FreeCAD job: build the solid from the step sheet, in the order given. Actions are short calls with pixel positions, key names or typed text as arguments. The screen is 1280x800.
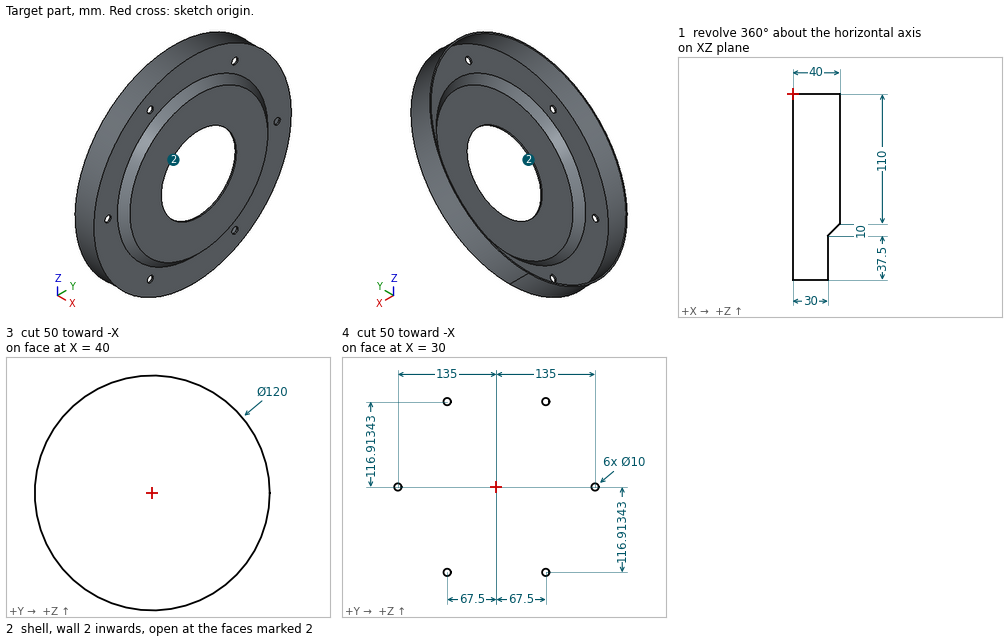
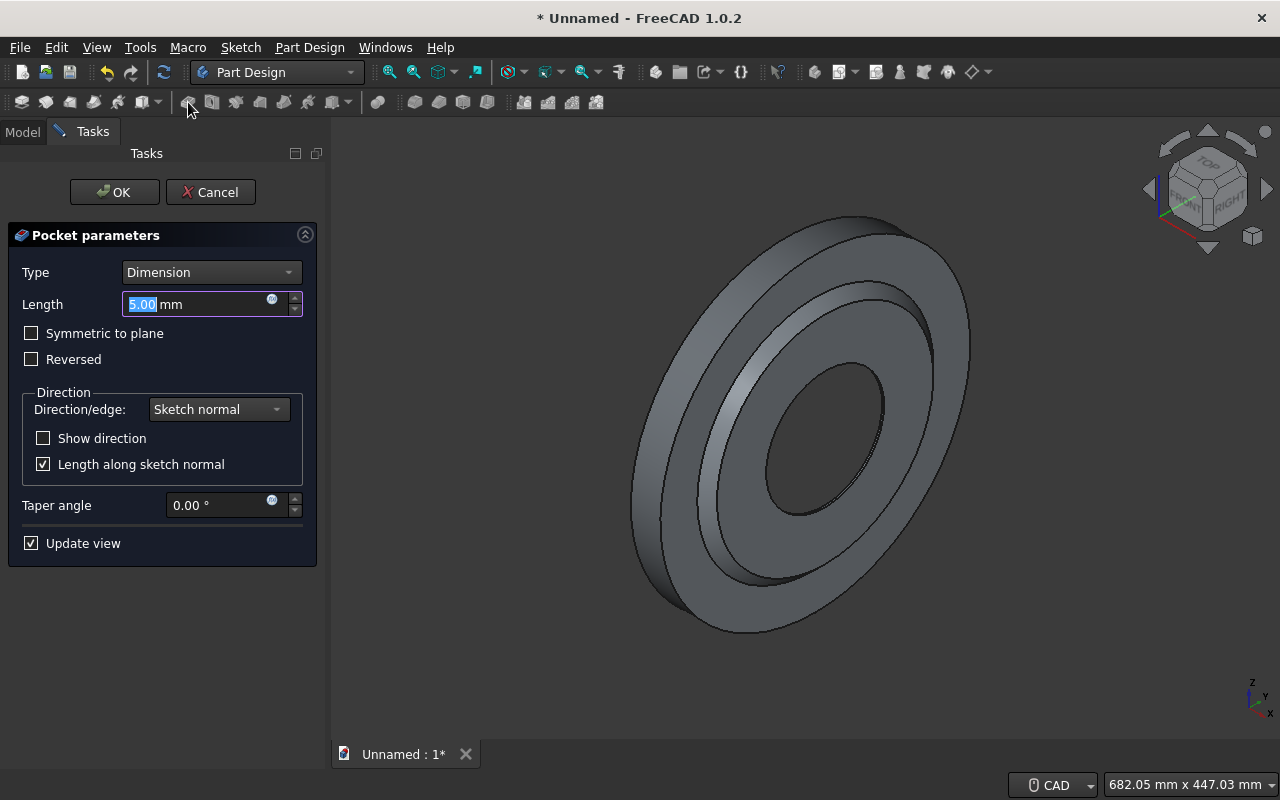
text(50)
key(Tab)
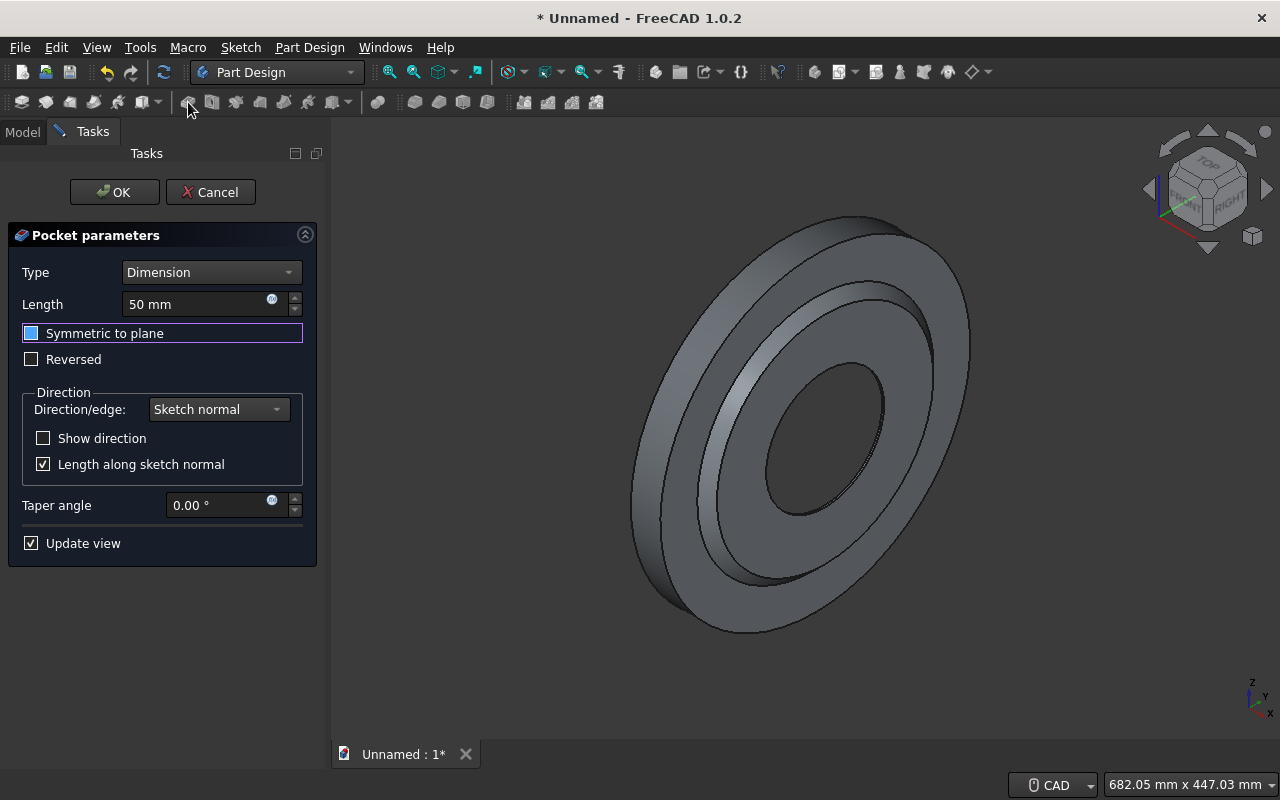
click(115, 192)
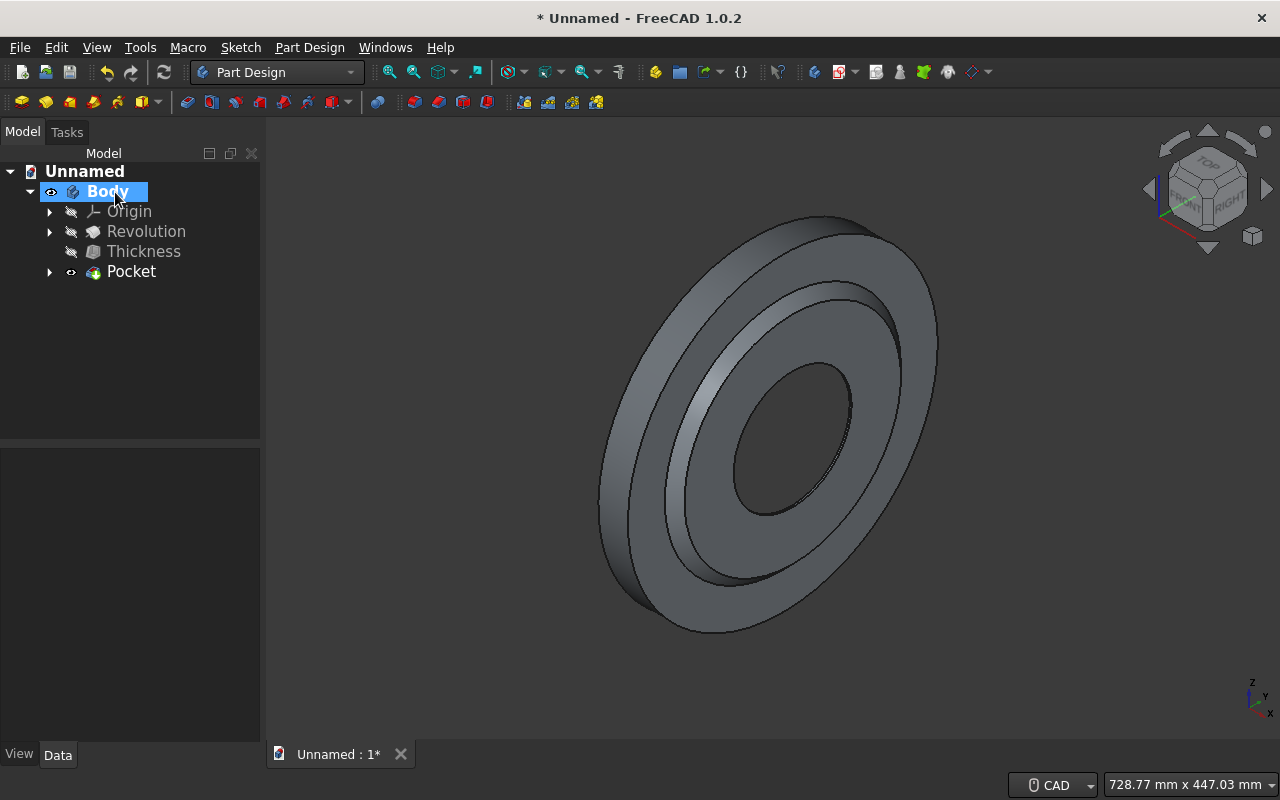
click(739, 611)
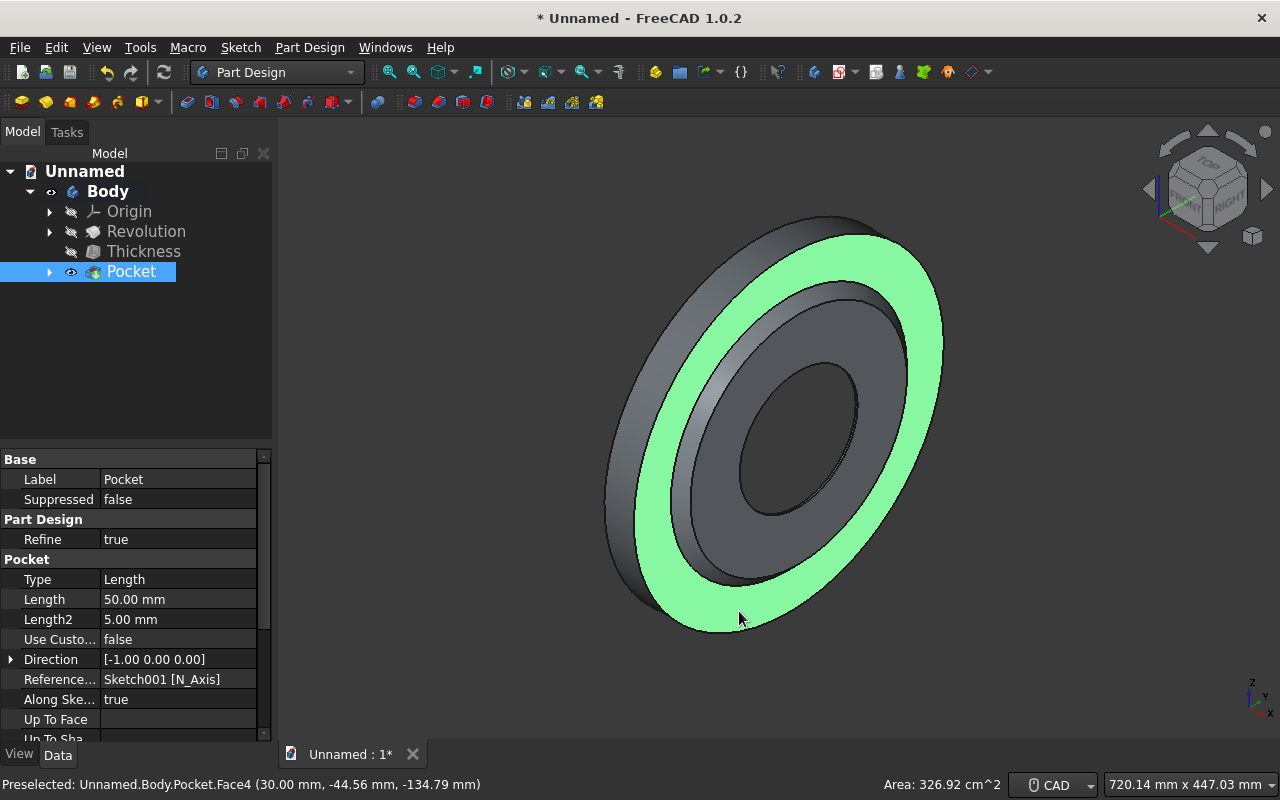
click(840, 72)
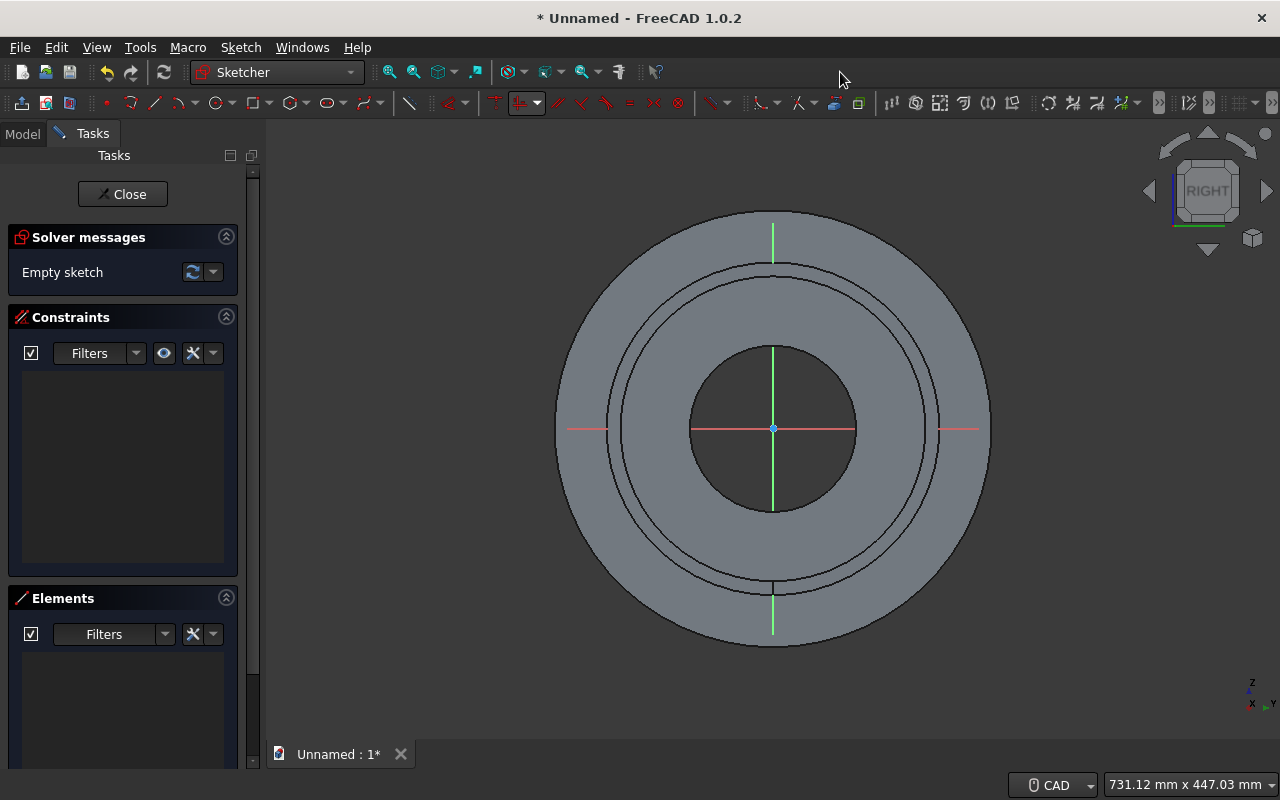
click(216, 104)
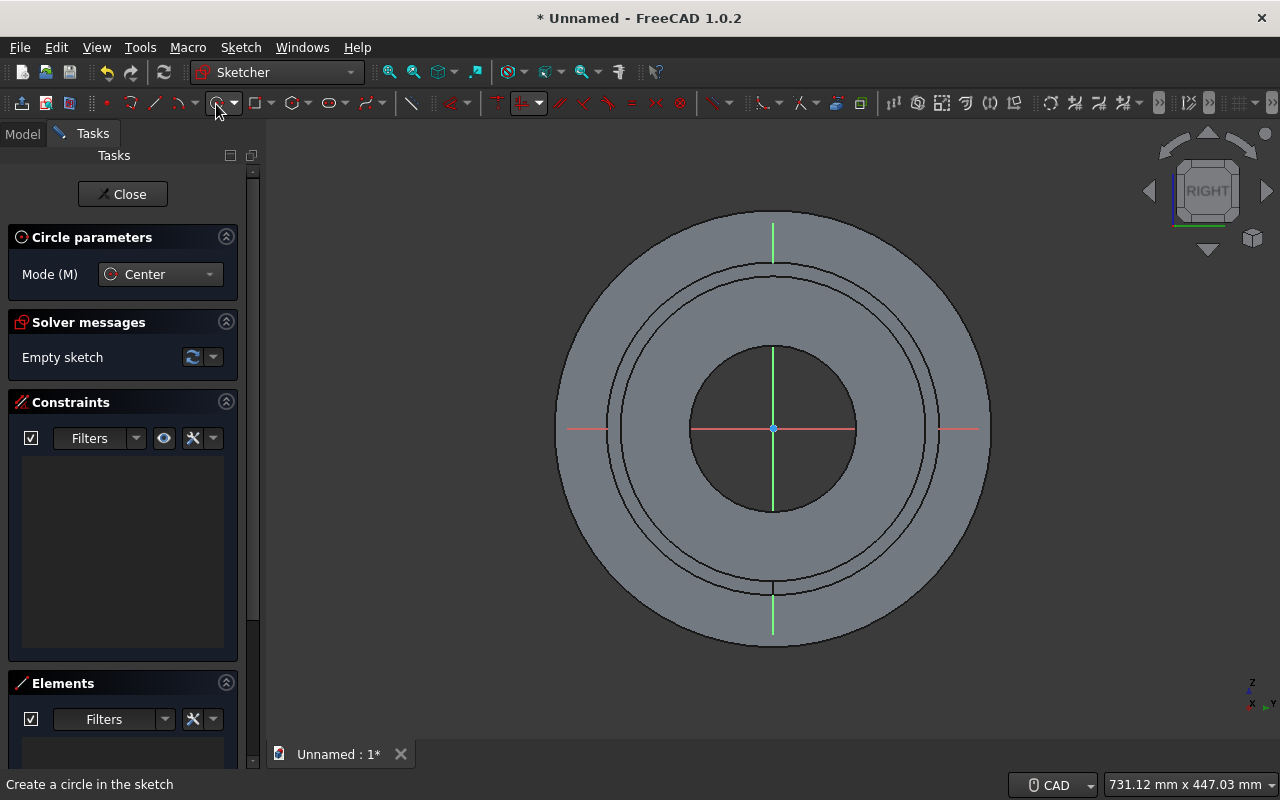
scroll(960, 429, up, 6)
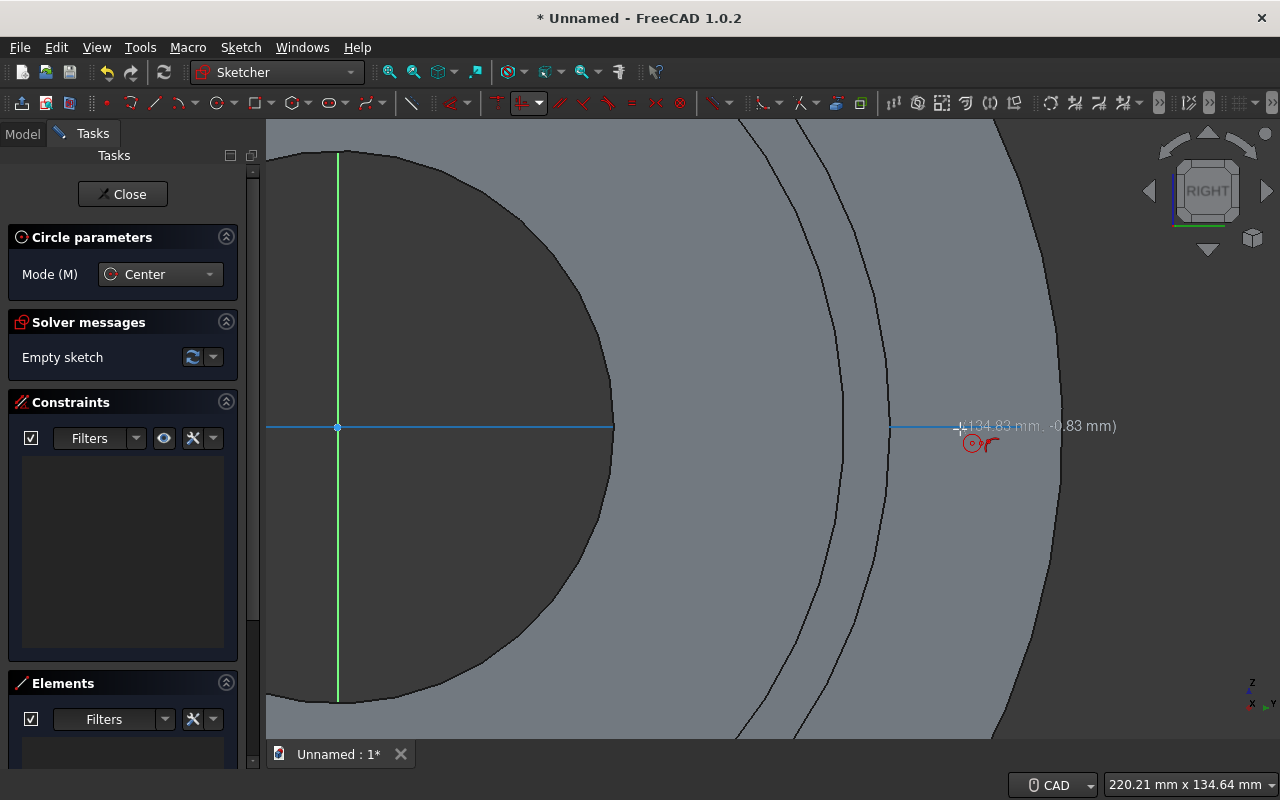
click(959, 427)
move(975, 411)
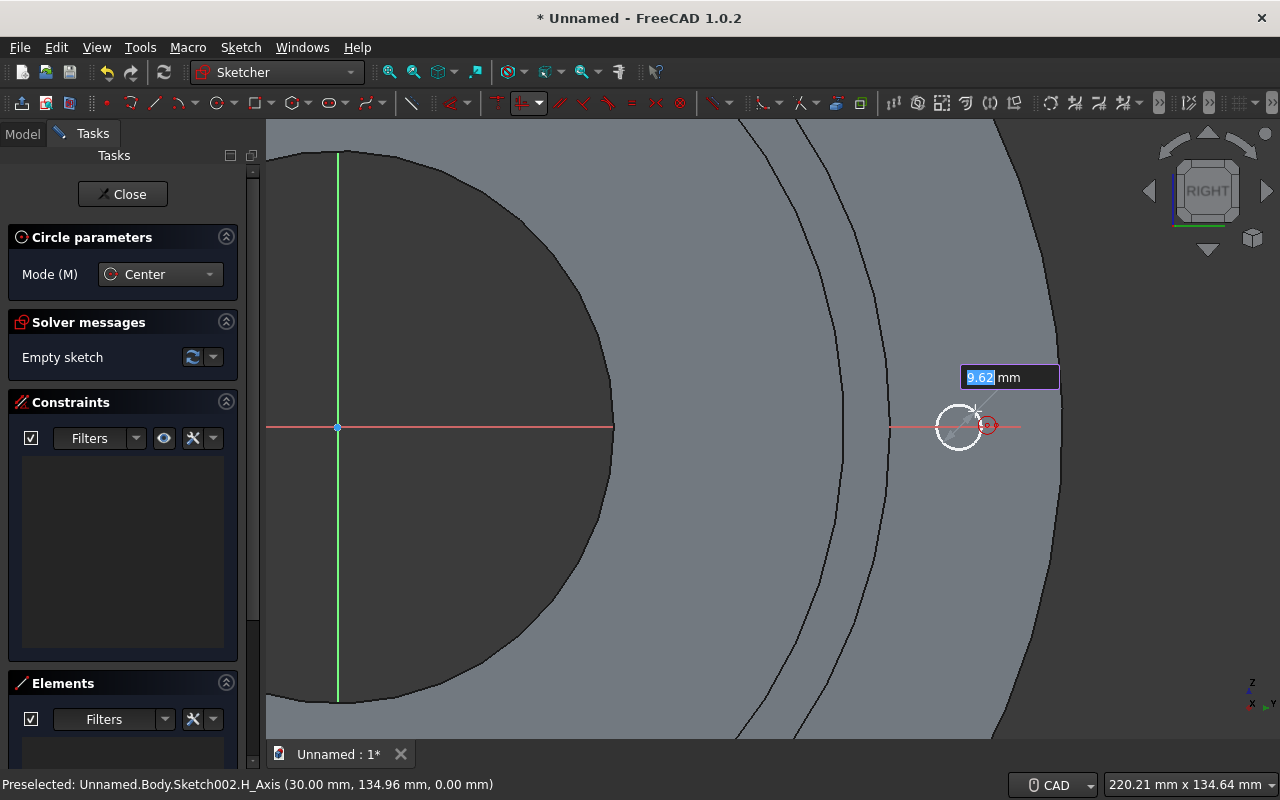
text(10)
key(Return)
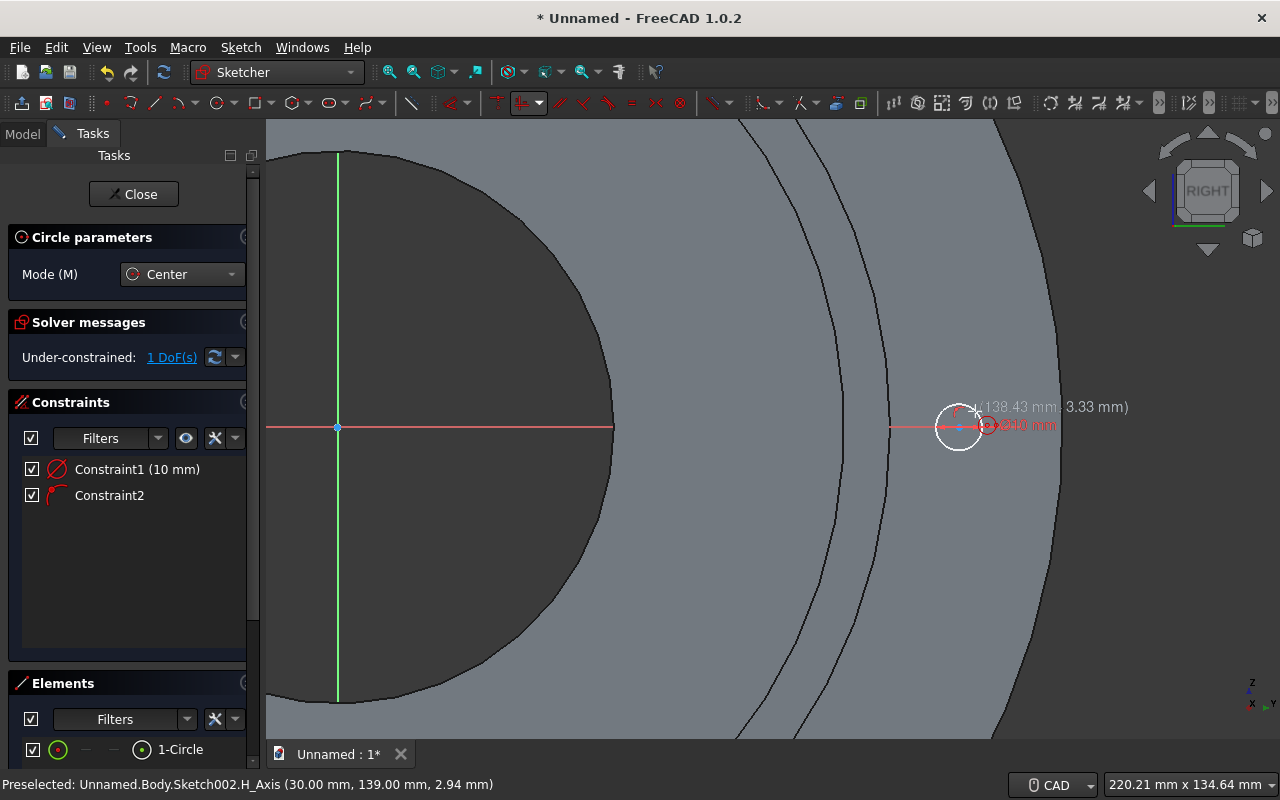
scroll(918, 430, down, 5)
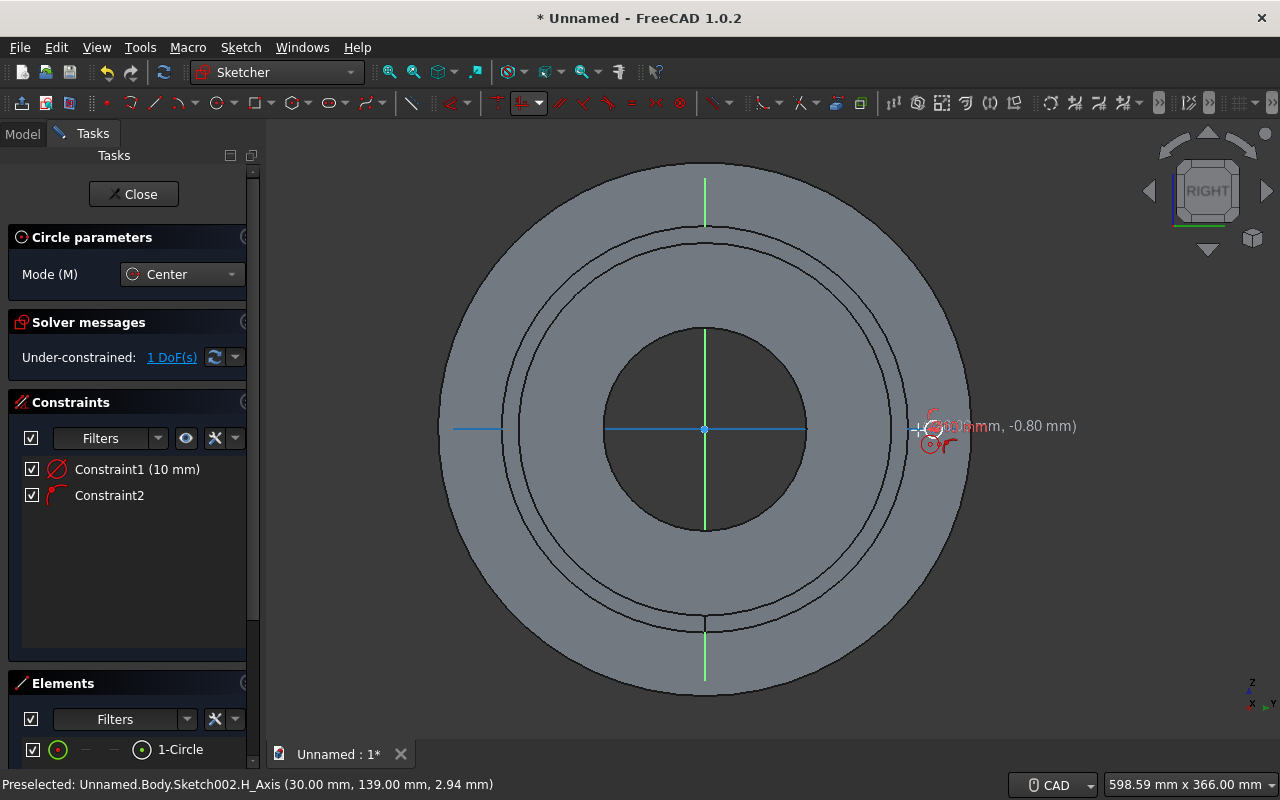
scroll(819, 627, up, 5)